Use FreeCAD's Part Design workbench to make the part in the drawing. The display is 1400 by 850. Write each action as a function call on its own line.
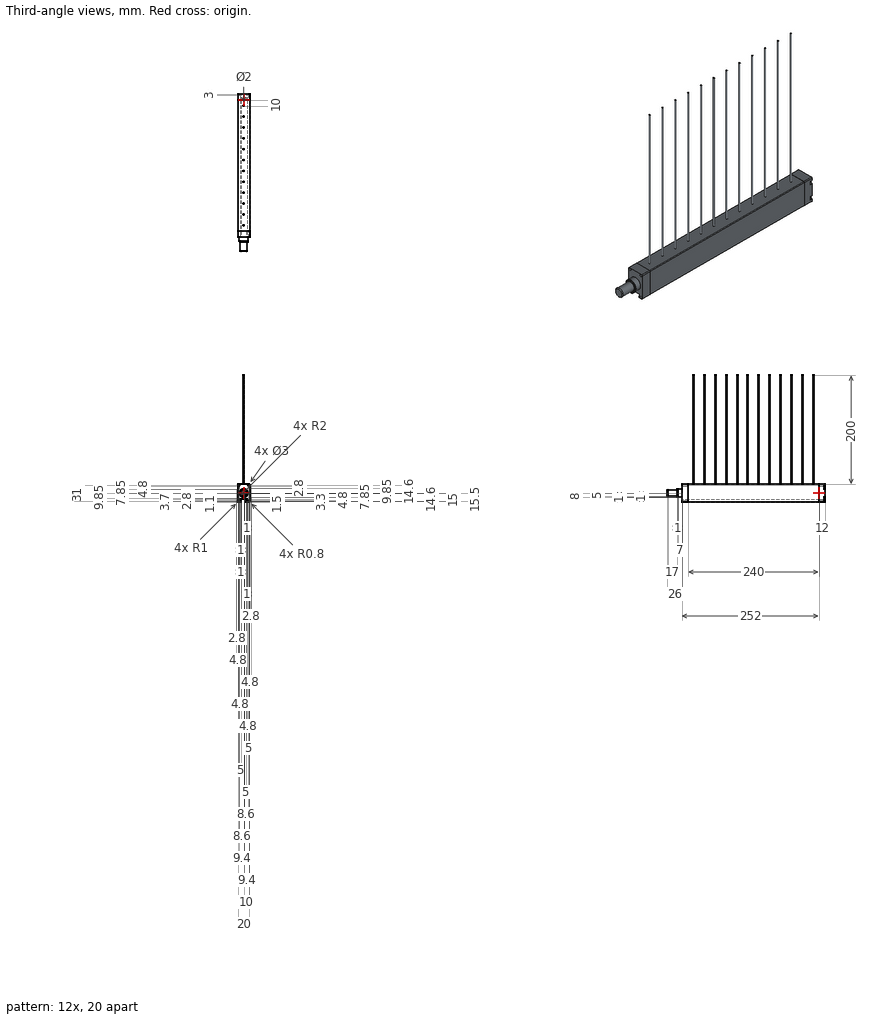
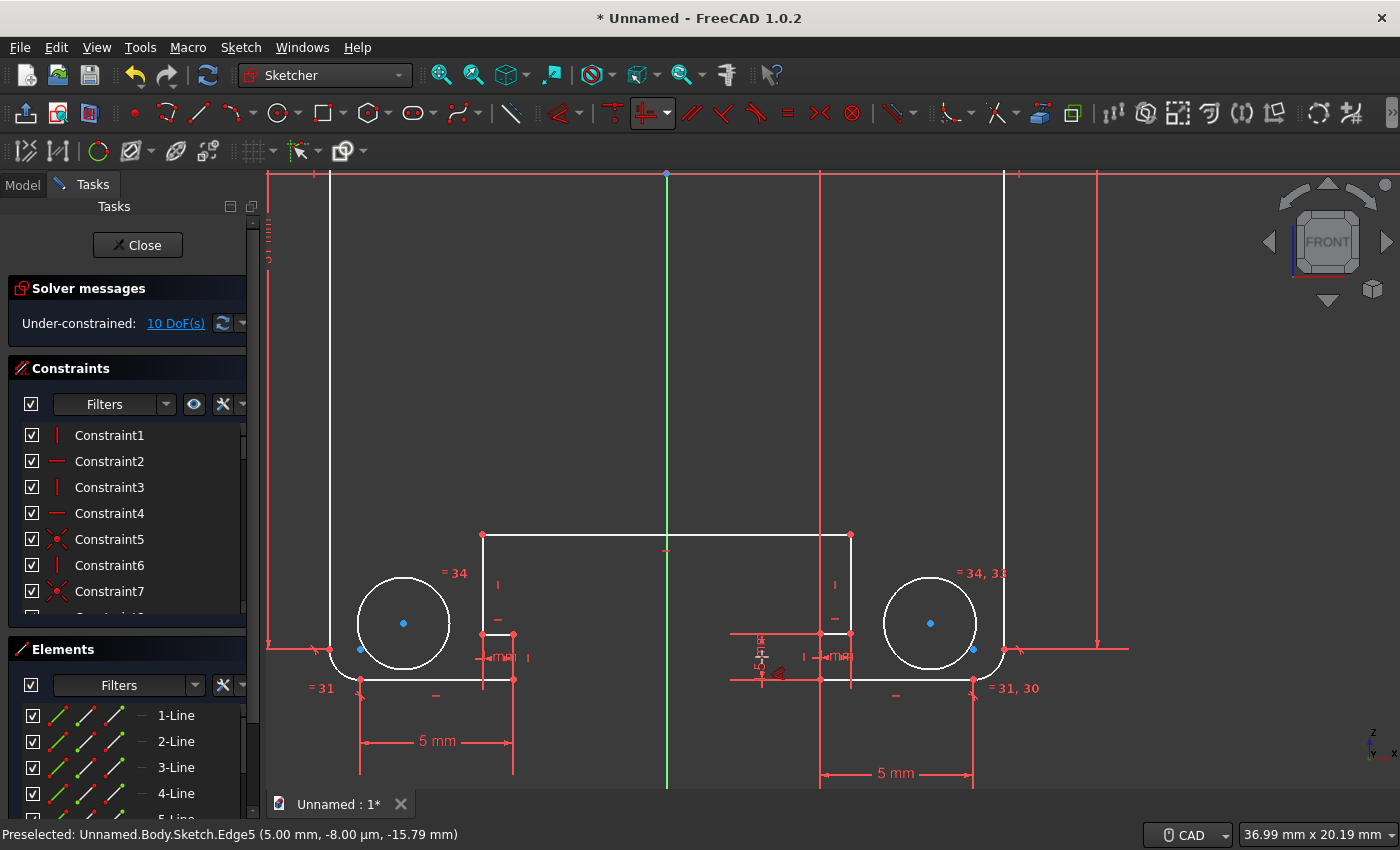
click(851, 604)
click(885, 584)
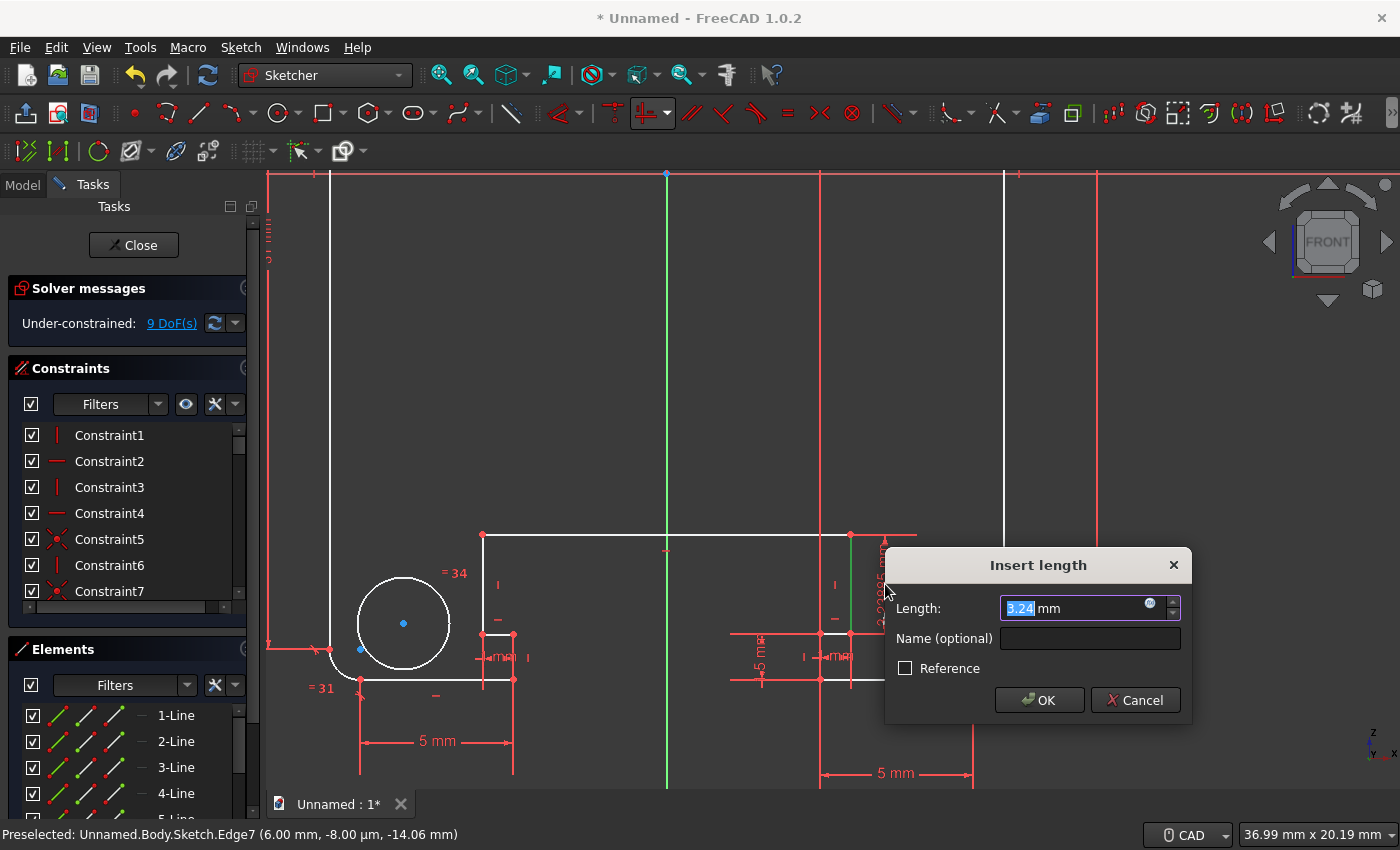
text(3.3)
key(Return)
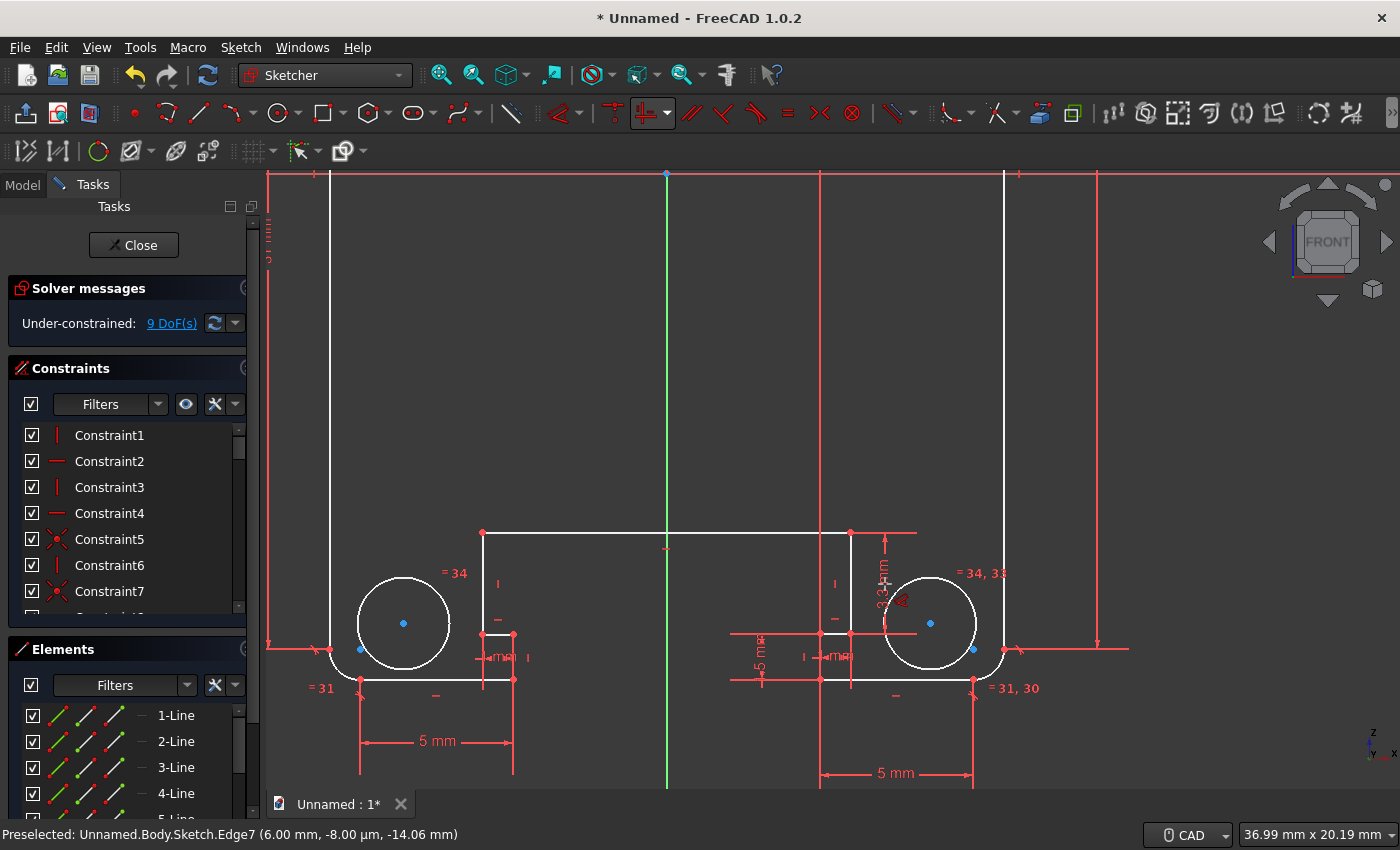
click(483, 563)
click(449, 584)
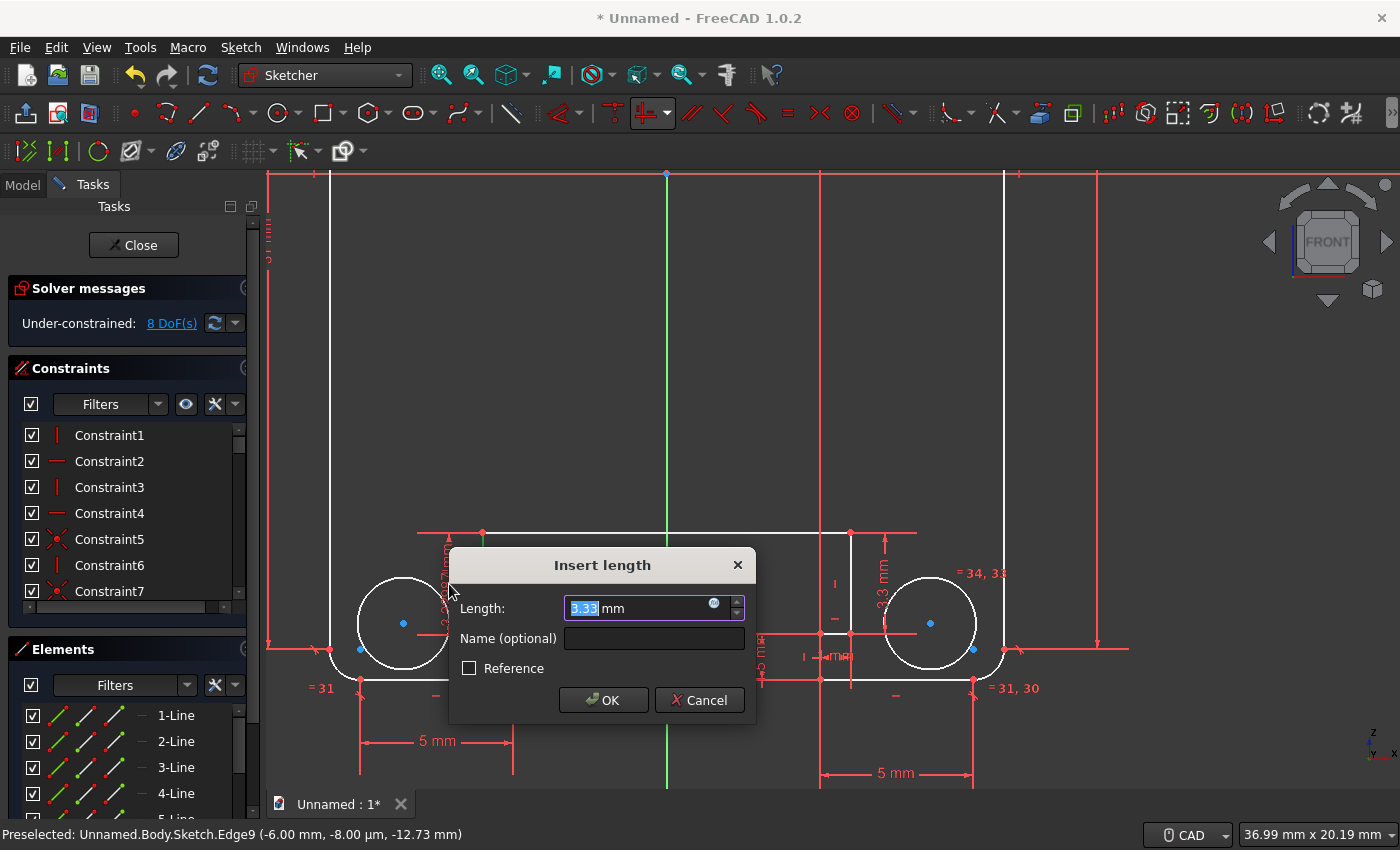
text(3.3)
key(Return)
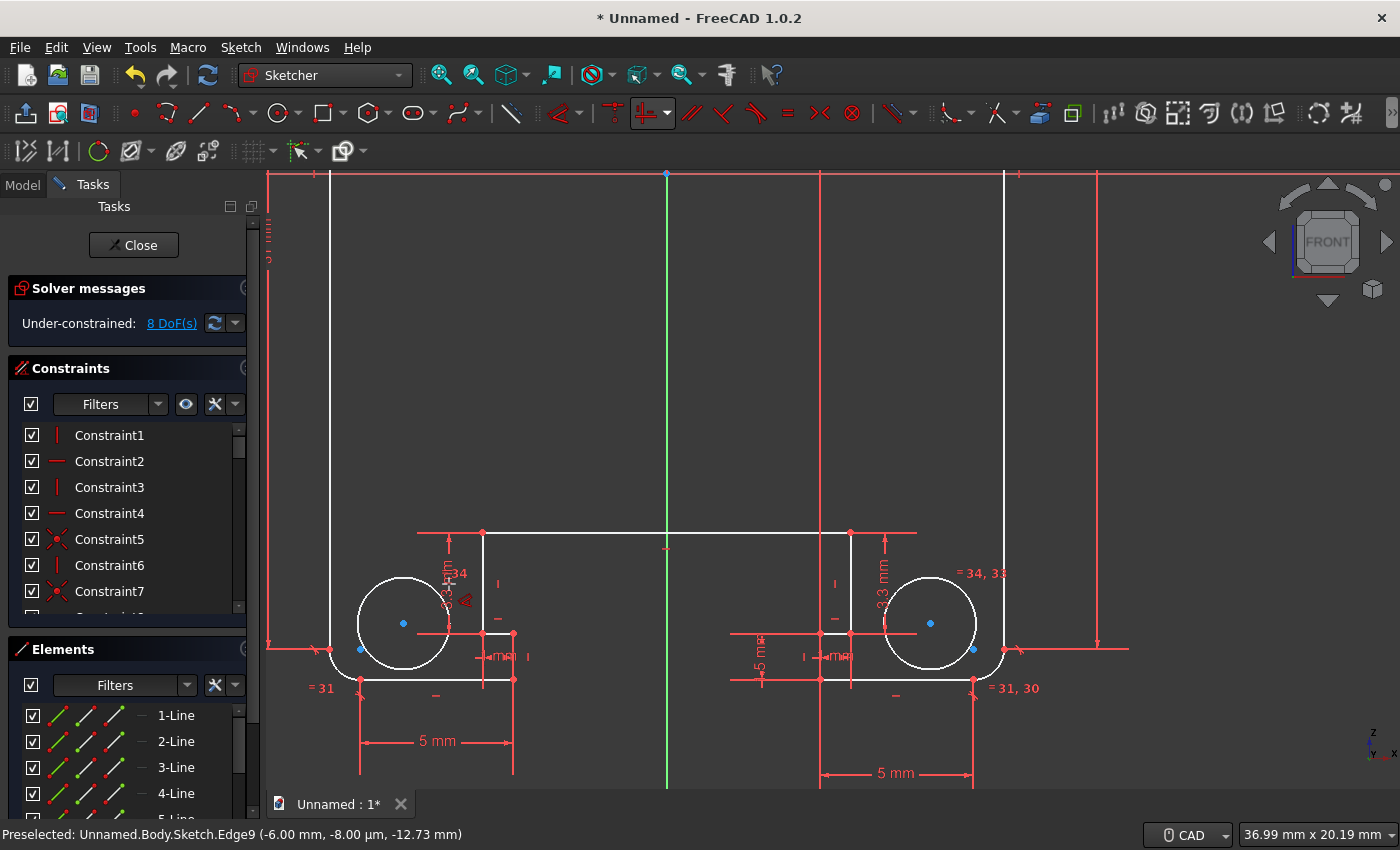
click(820, 634)
click(854, 416)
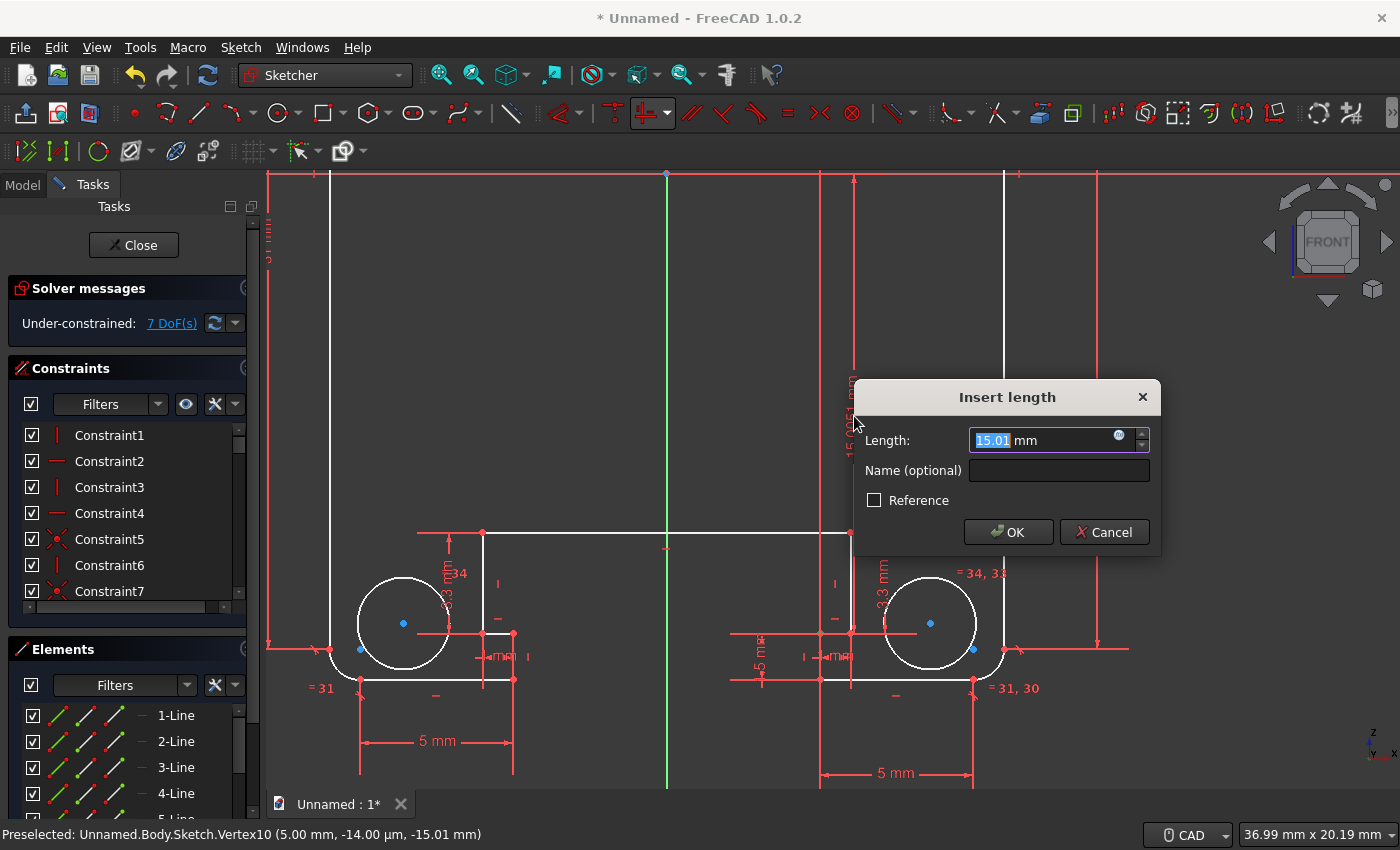
text(15)
key(Return)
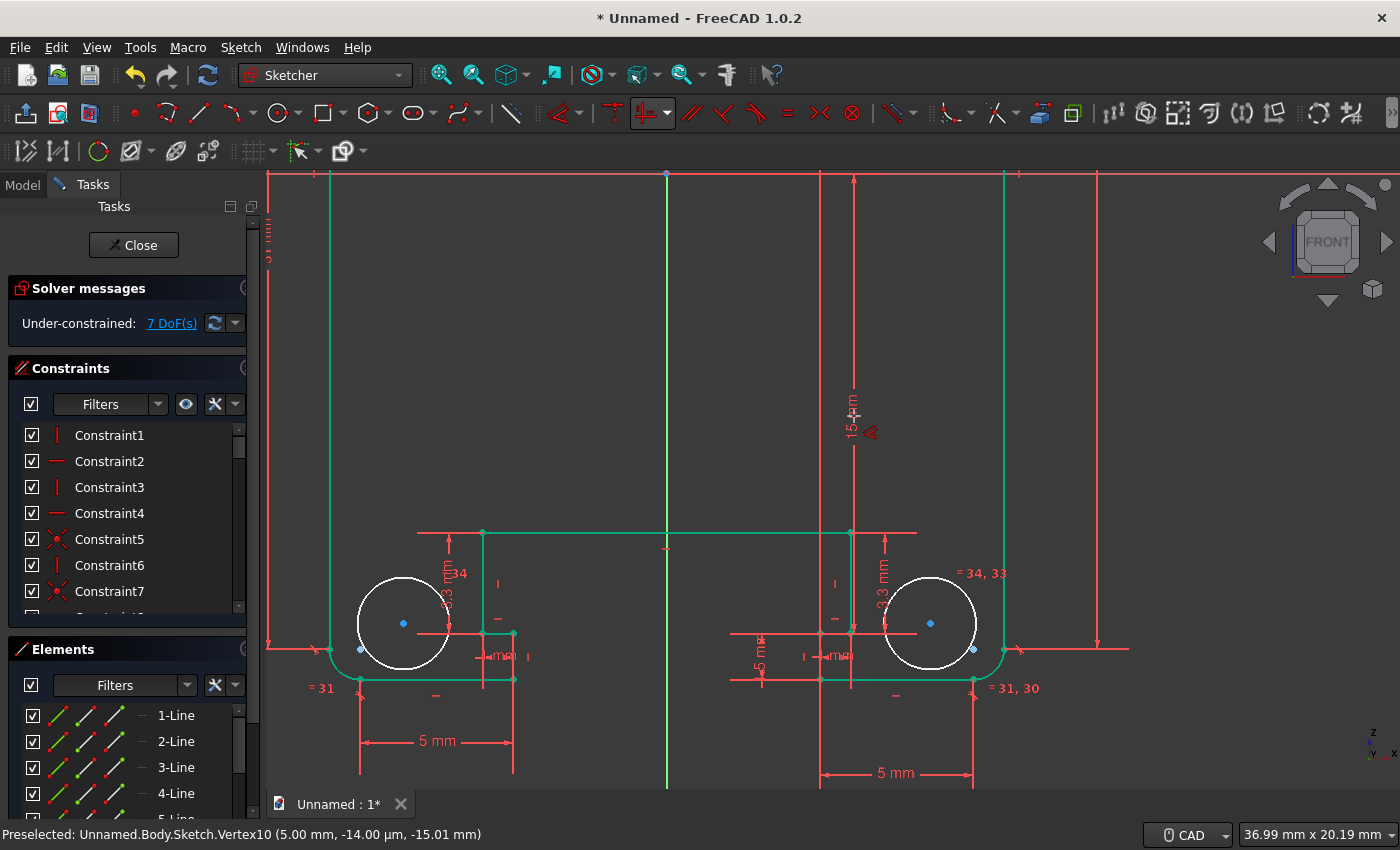
scroll(821, 657, down, 5)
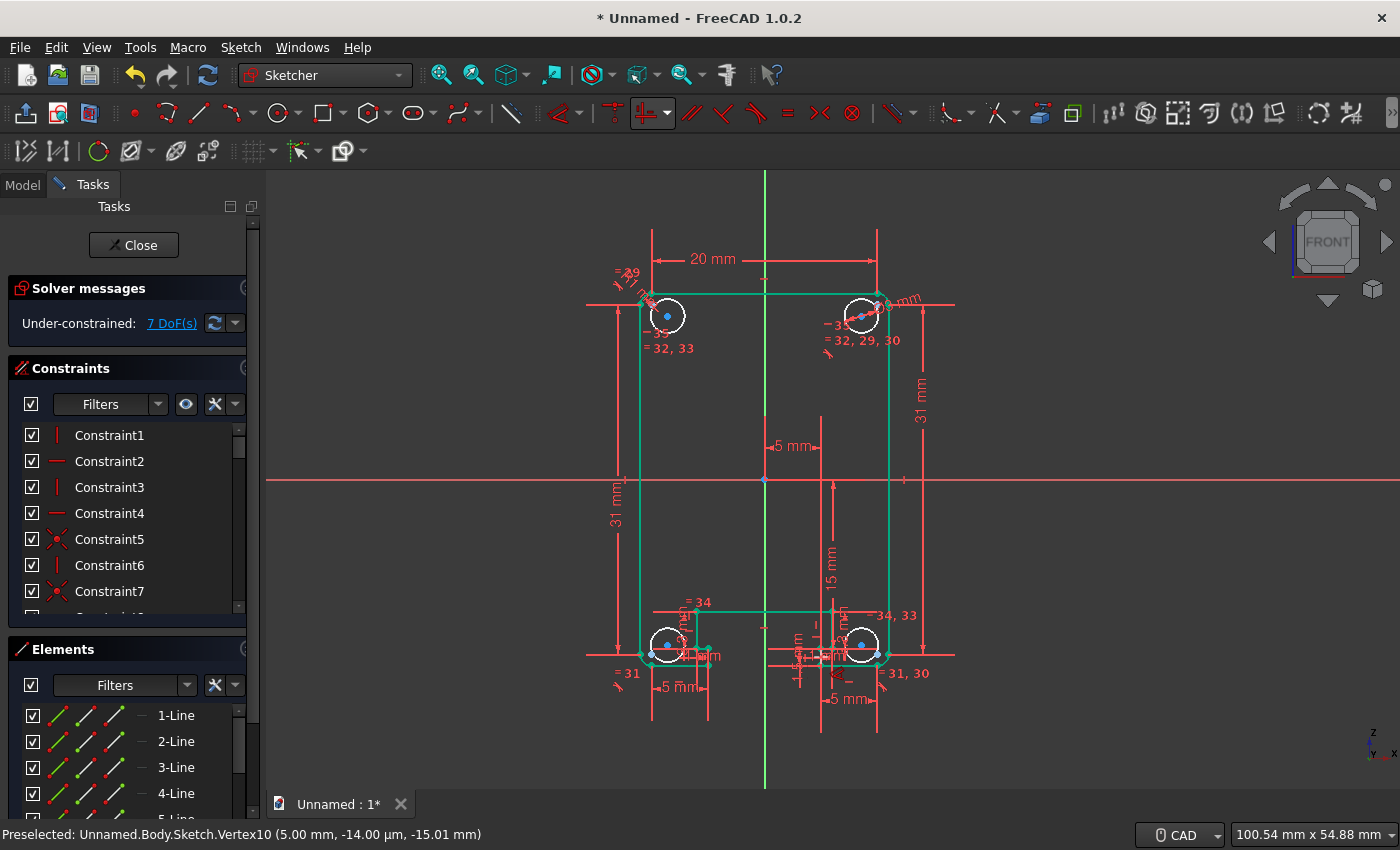
click(861, 316)
click(813, 514)